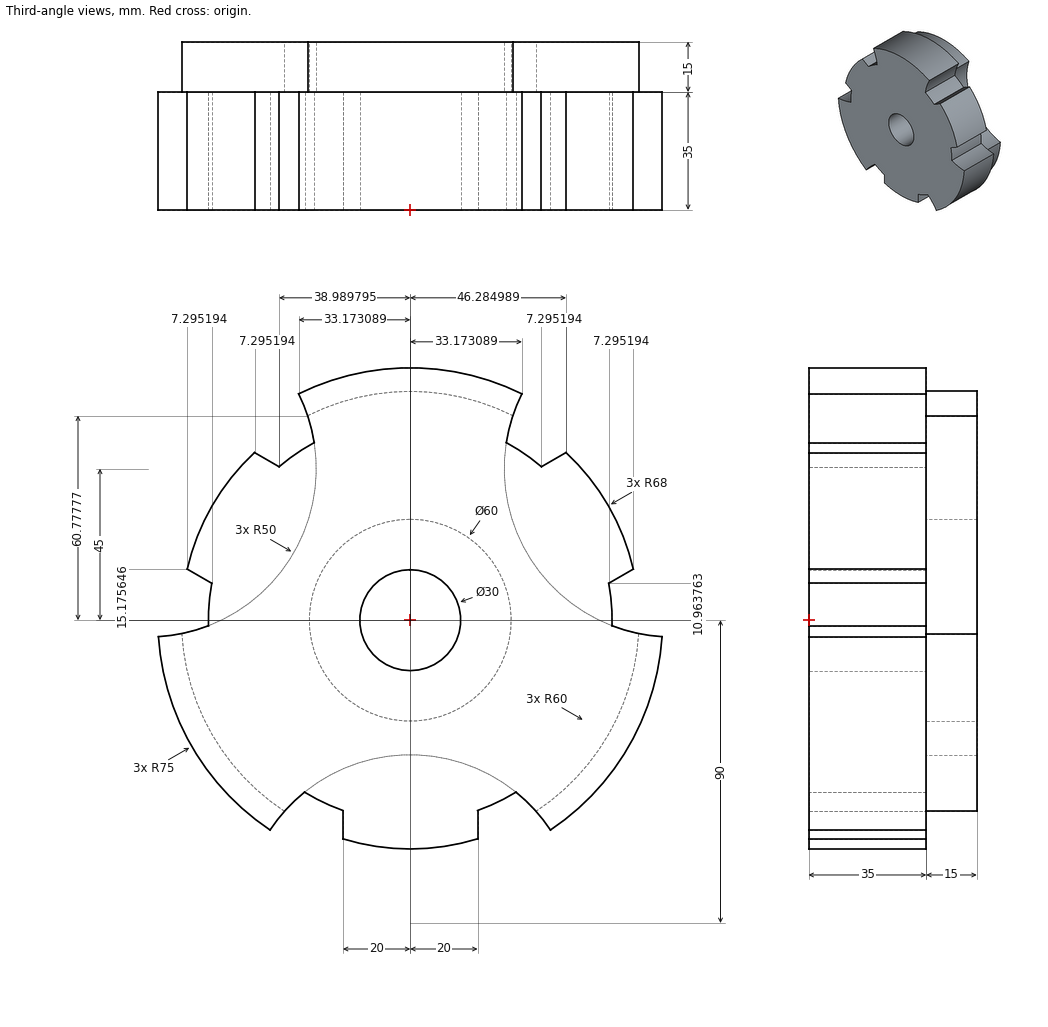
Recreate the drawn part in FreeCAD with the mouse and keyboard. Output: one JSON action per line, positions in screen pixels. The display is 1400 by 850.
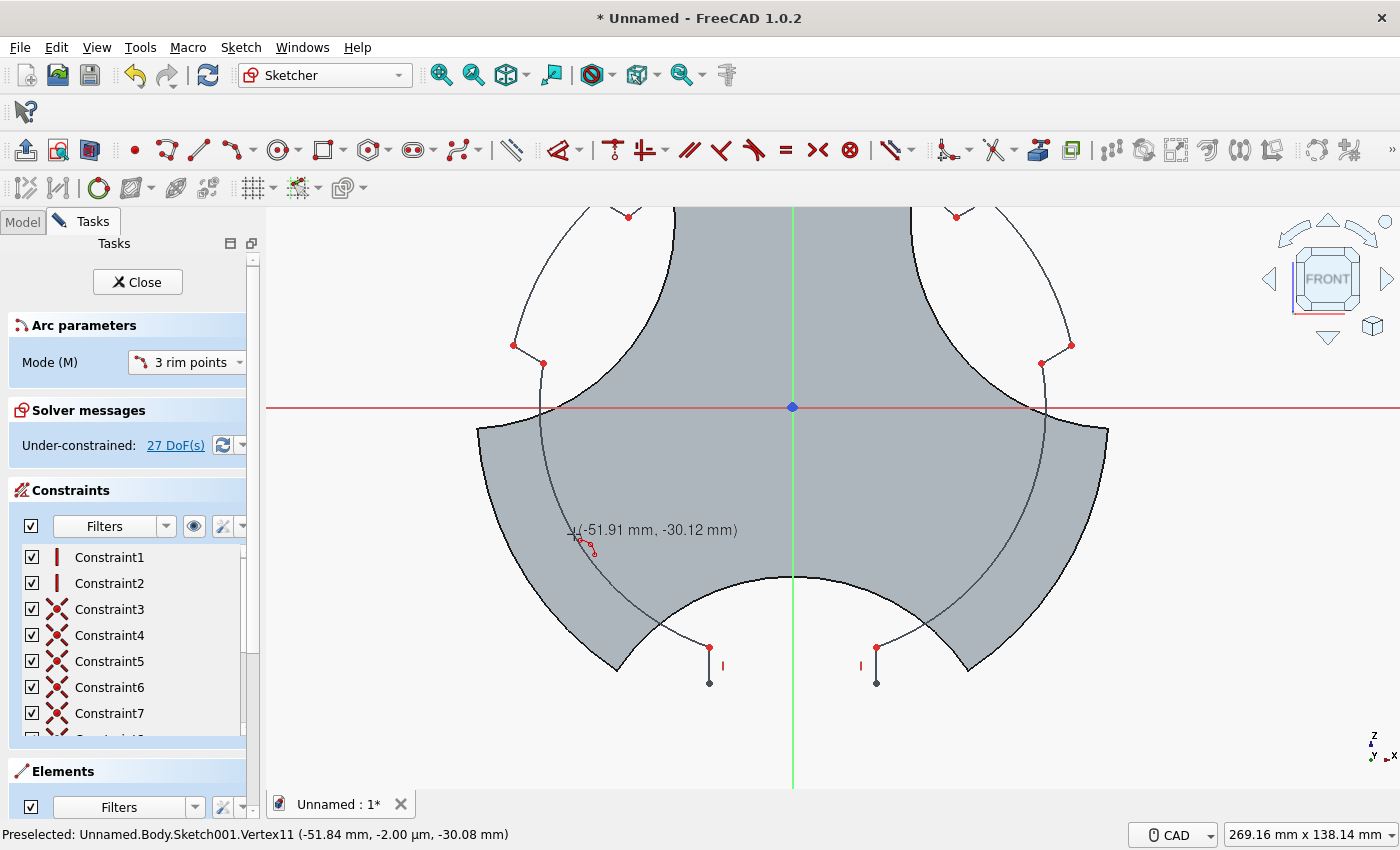
{"action": "left_click", "coordinate": [709, 683]}
{"action": "left_click", "coordinate": [876, 683]}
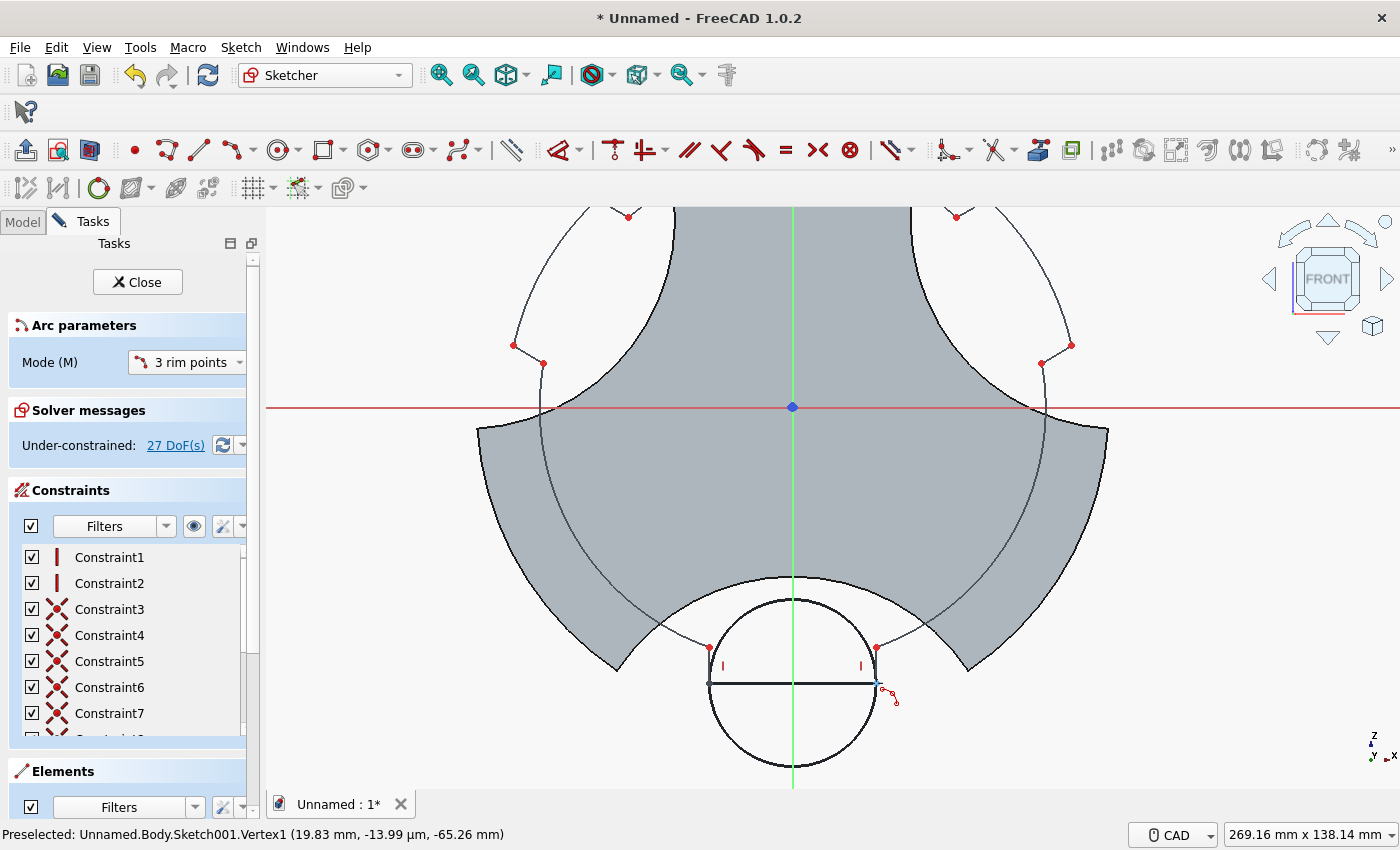
{"action": "scroll", "coordinate": [776, 694], "scroll_direction": "up", "scroll_amount": 2}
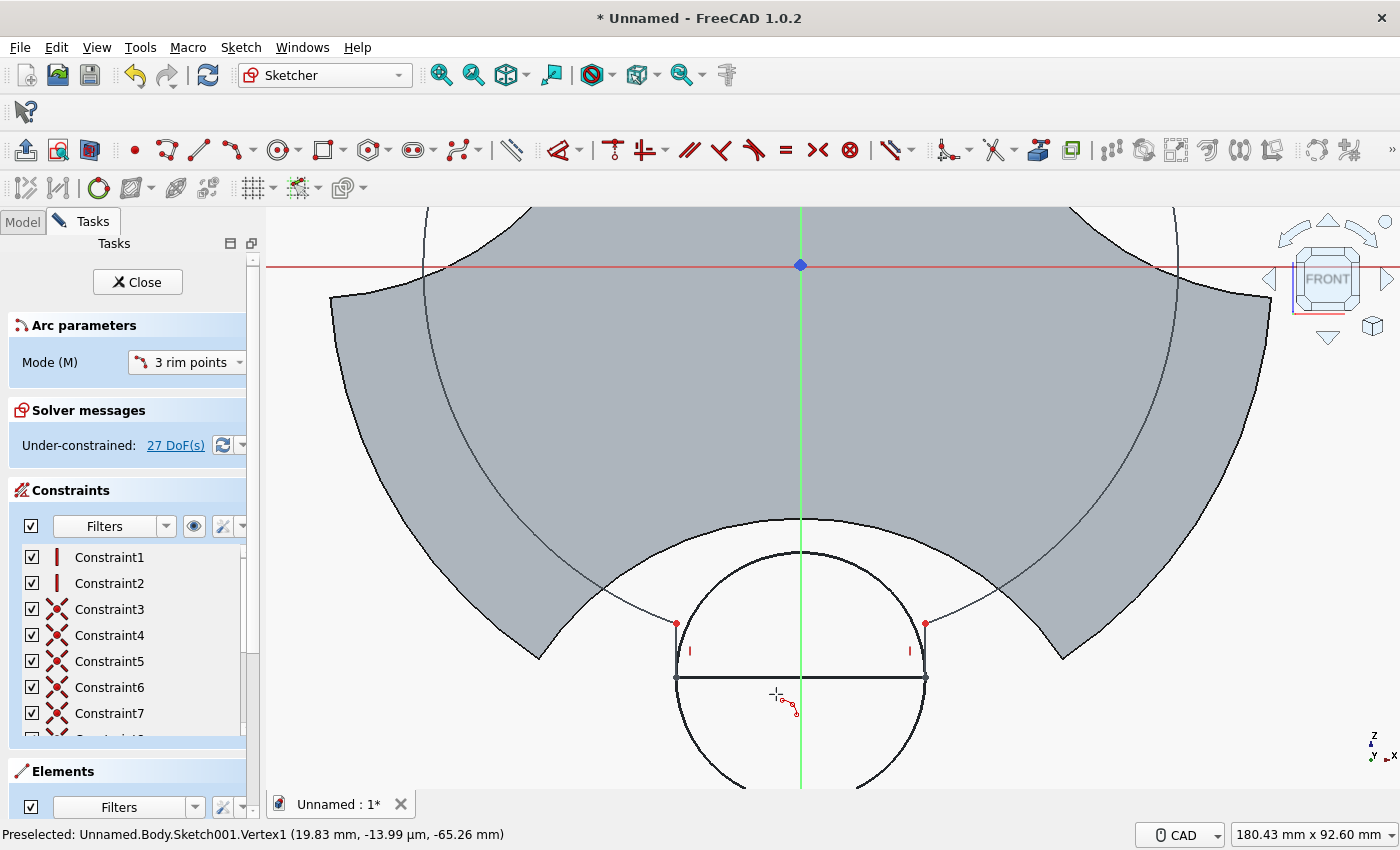
{"action": "left_click", "coordinate": [775, 694]}
{"action": "key", "text": "Escape"}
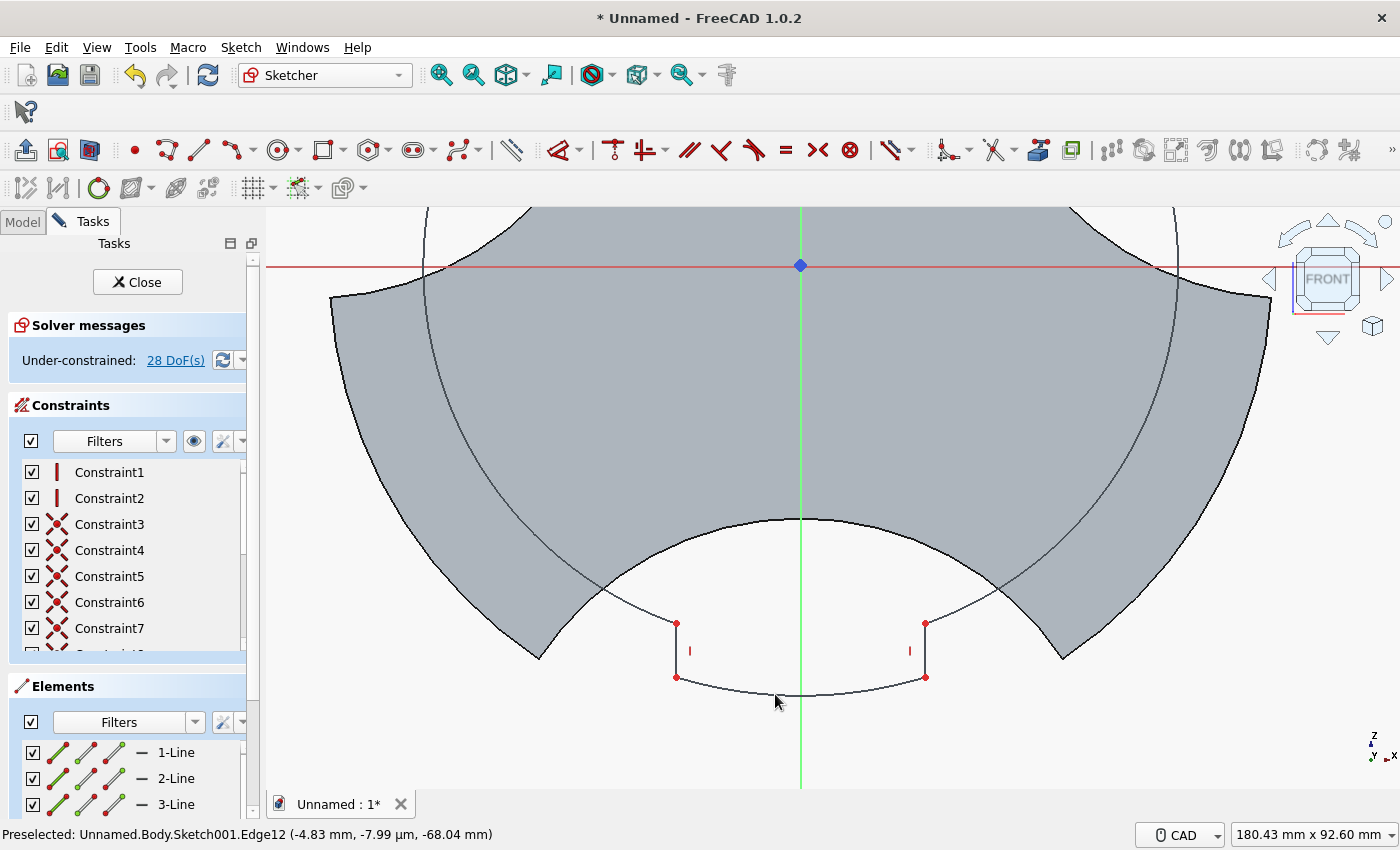
{"action": "left_click", "coordinate": [1061, 541]}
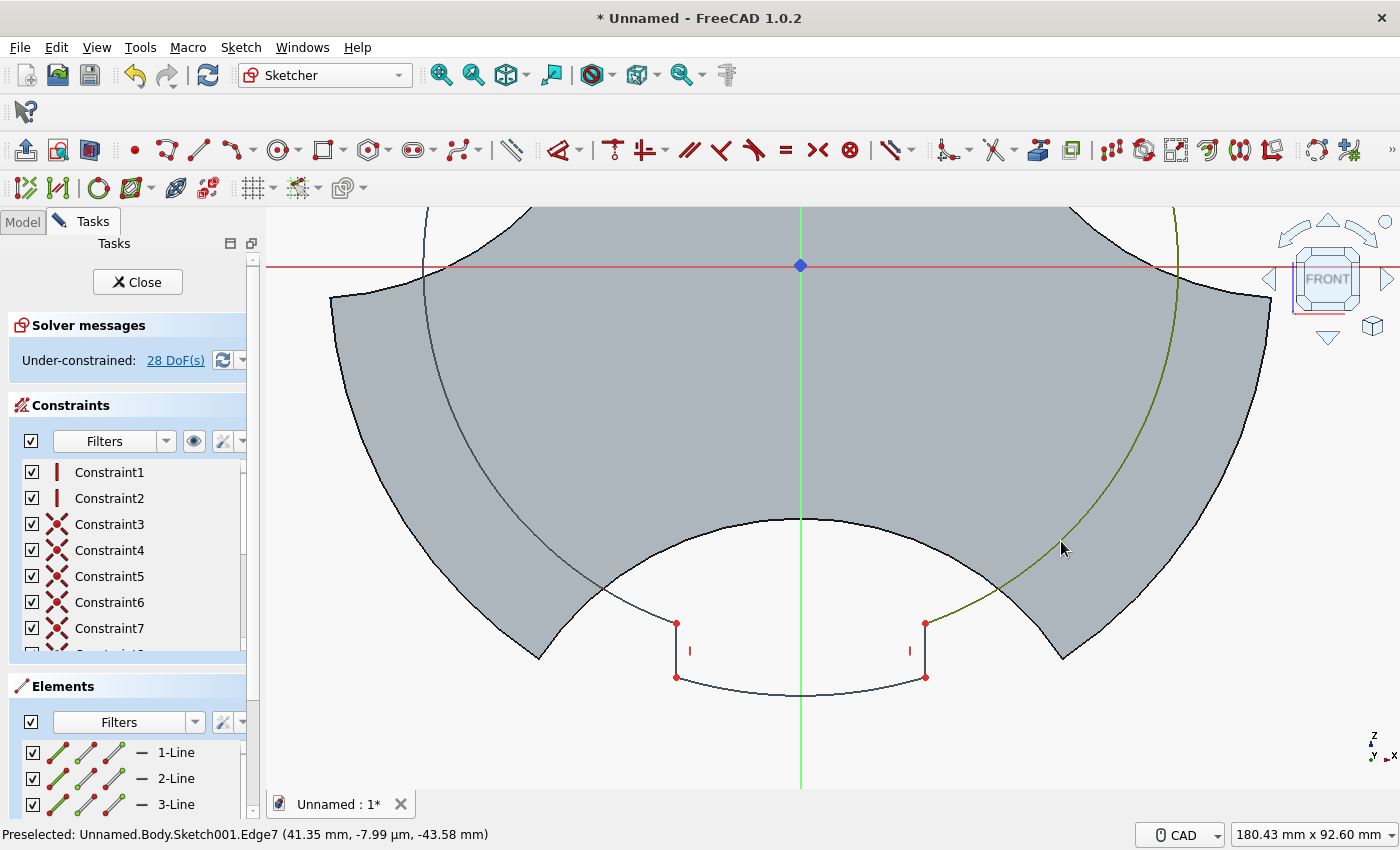
{"action": "scroll", "coordinate": [735, 666], "scroll_direction": "down", "scroll_amount": 4}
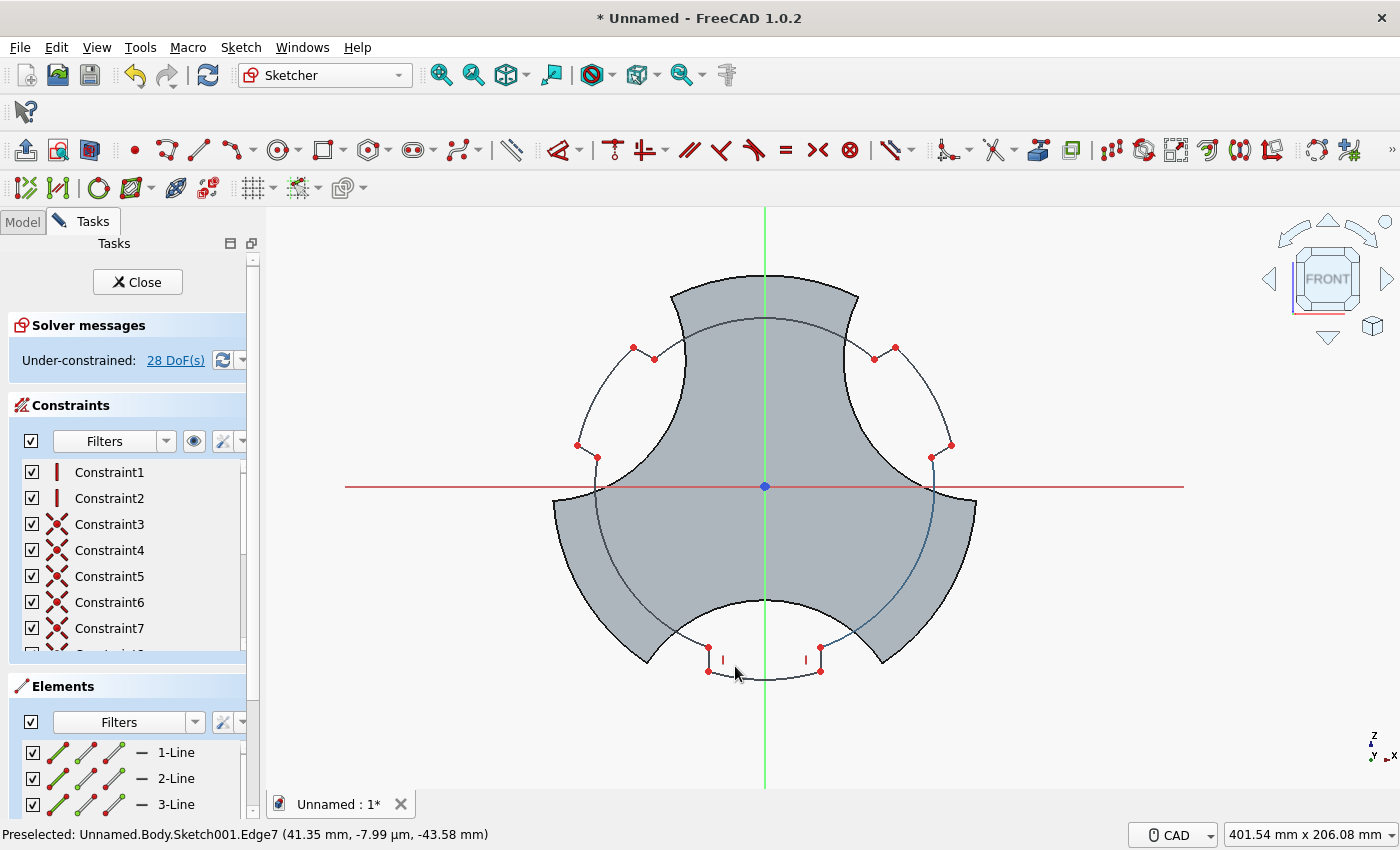
{"action": "left_click", "coordinate": [941, 413]}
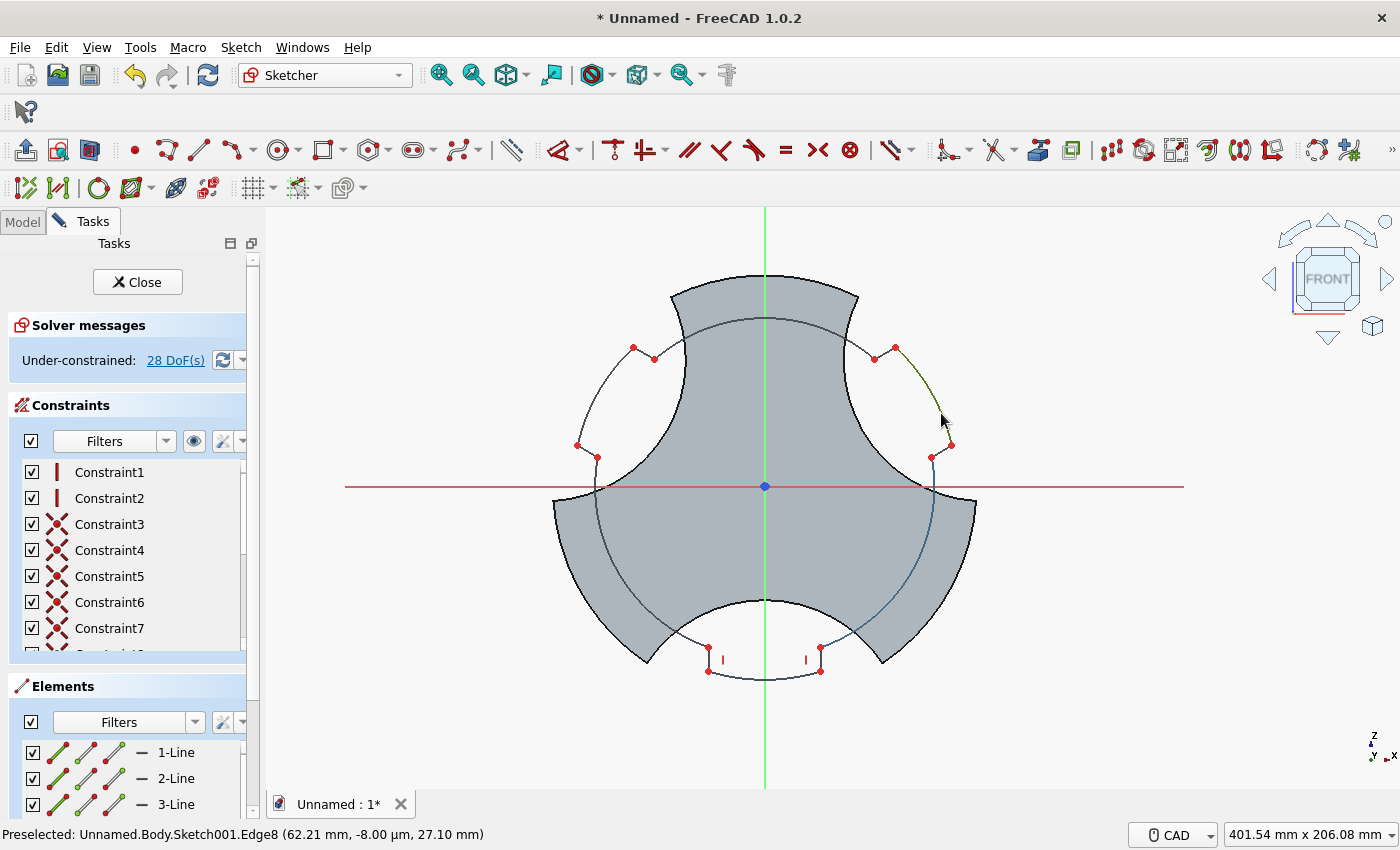
{"action": "left_click", "coordinate": [614, 150]}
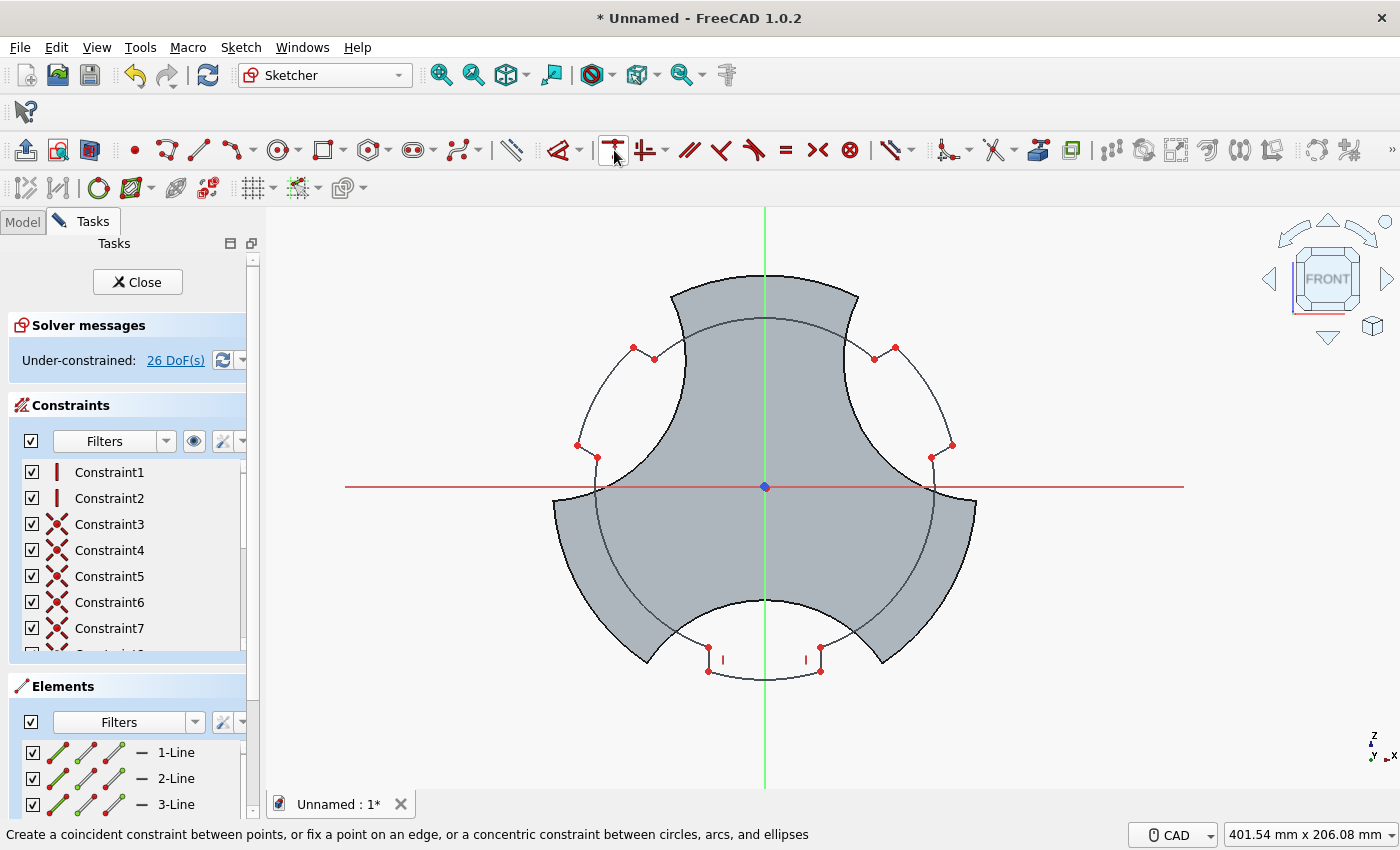
{"action": "left_click", "coordinate": [882, 611]}